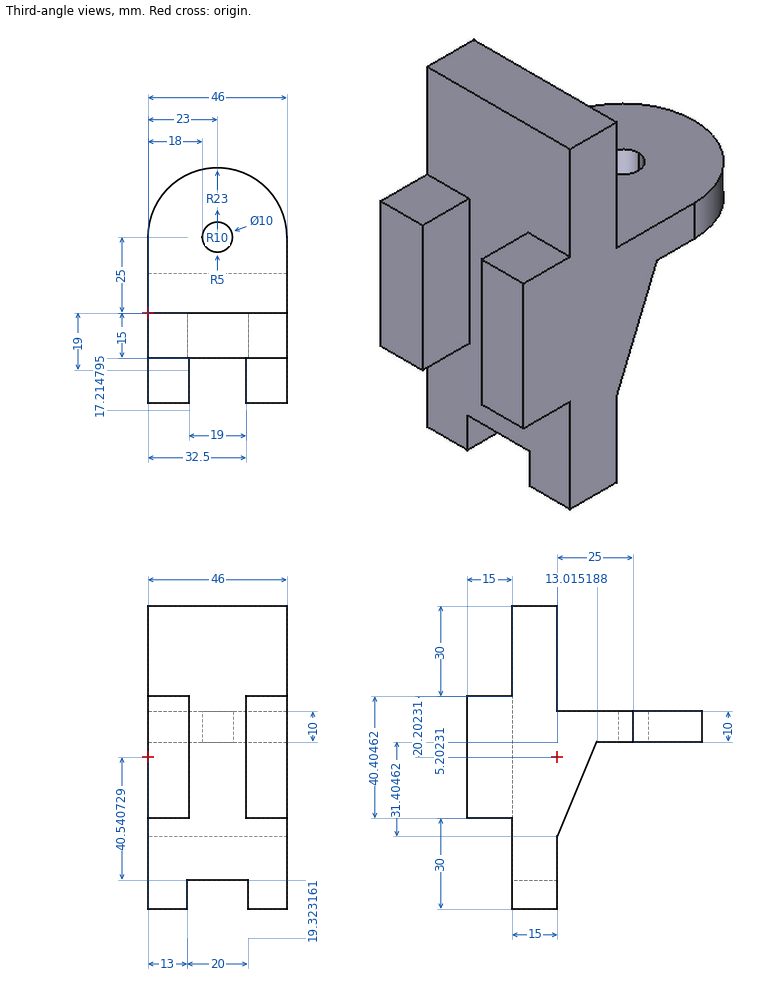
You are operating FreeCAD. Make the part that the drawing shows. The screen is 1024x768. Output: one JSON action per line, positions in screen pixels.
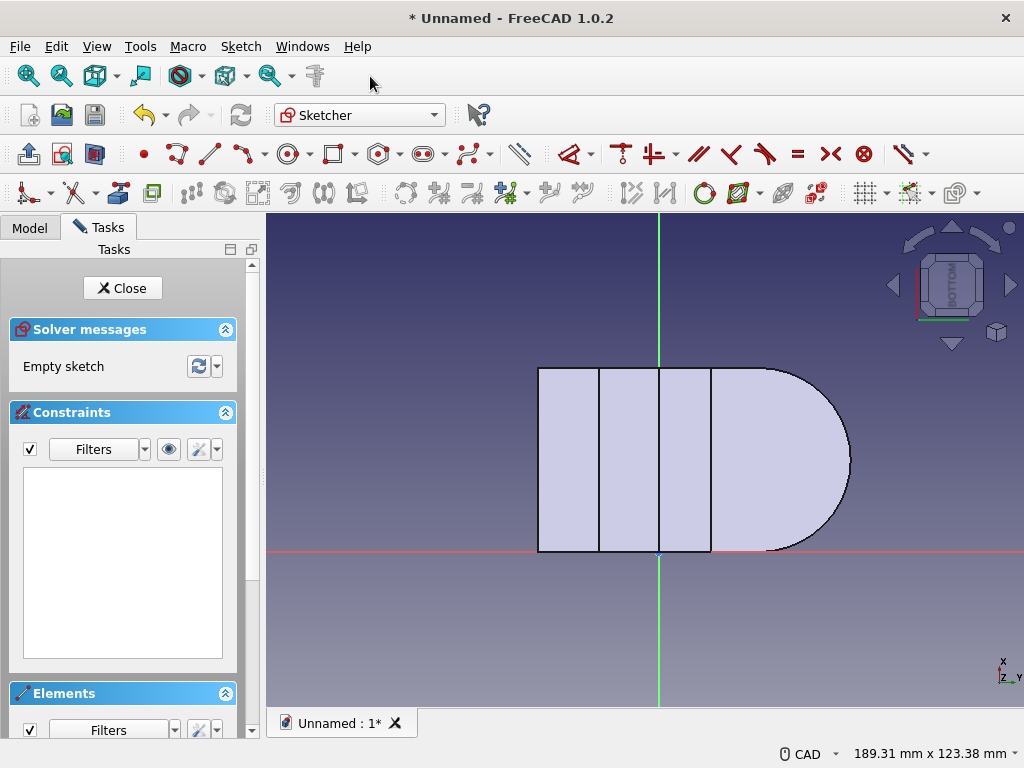
{"action": "key", "text": "q s"}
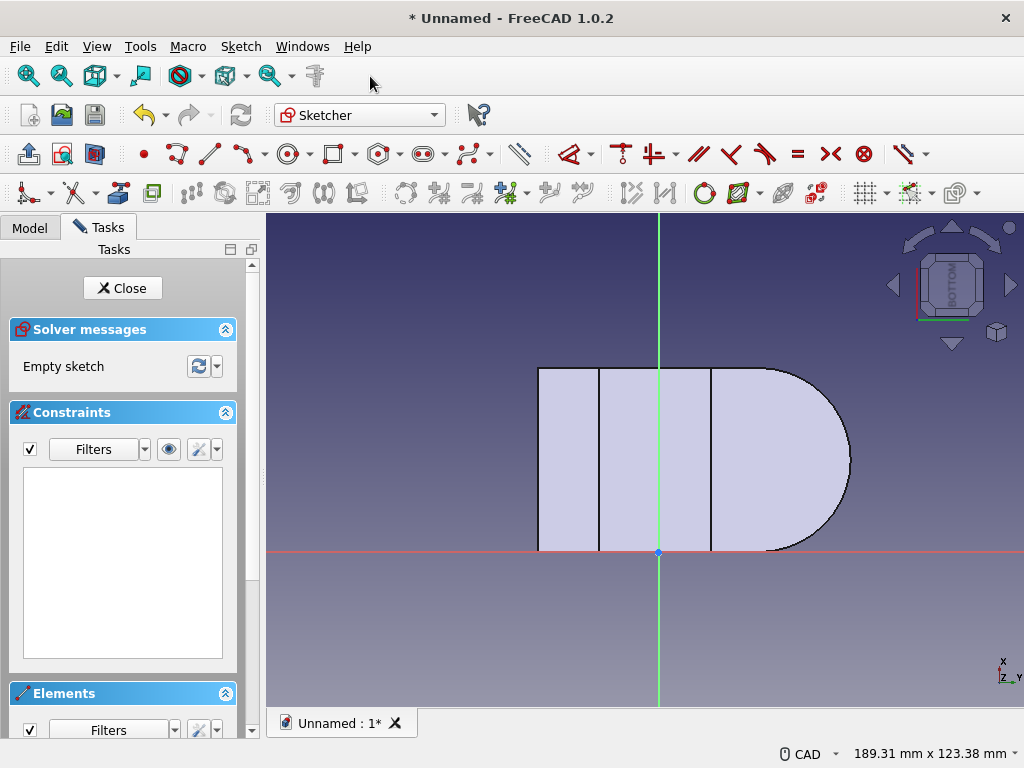
{"action": "scroll", "coordinate": [787, 460], "scroll_direction": "up", "scroll_amount": 10}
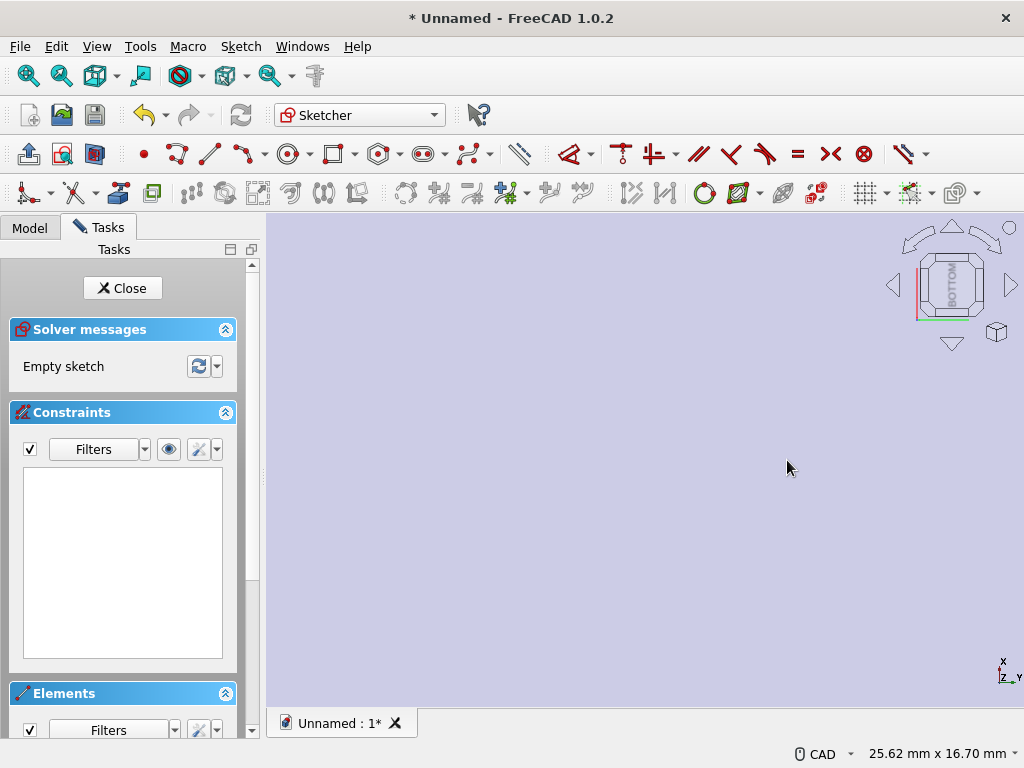
{"action": "key", "text": "g c"}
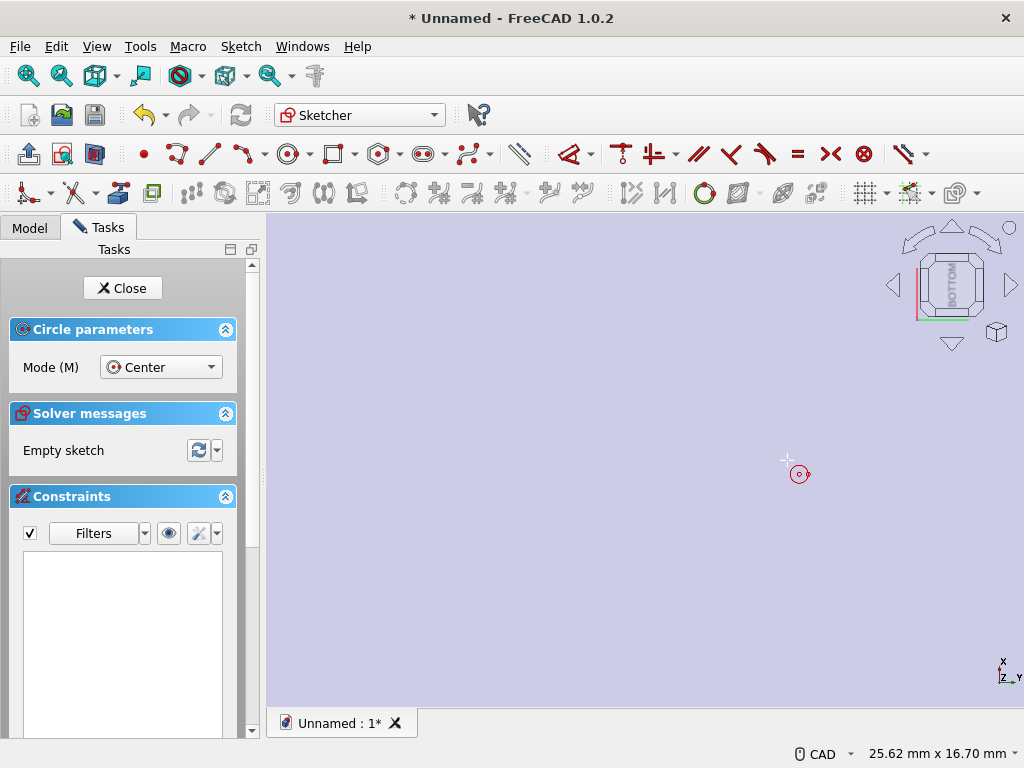
{"action": "left_click", "coordinate": [573, 457]}
{"action": "mouse_move", "coordinate": [678, 352]}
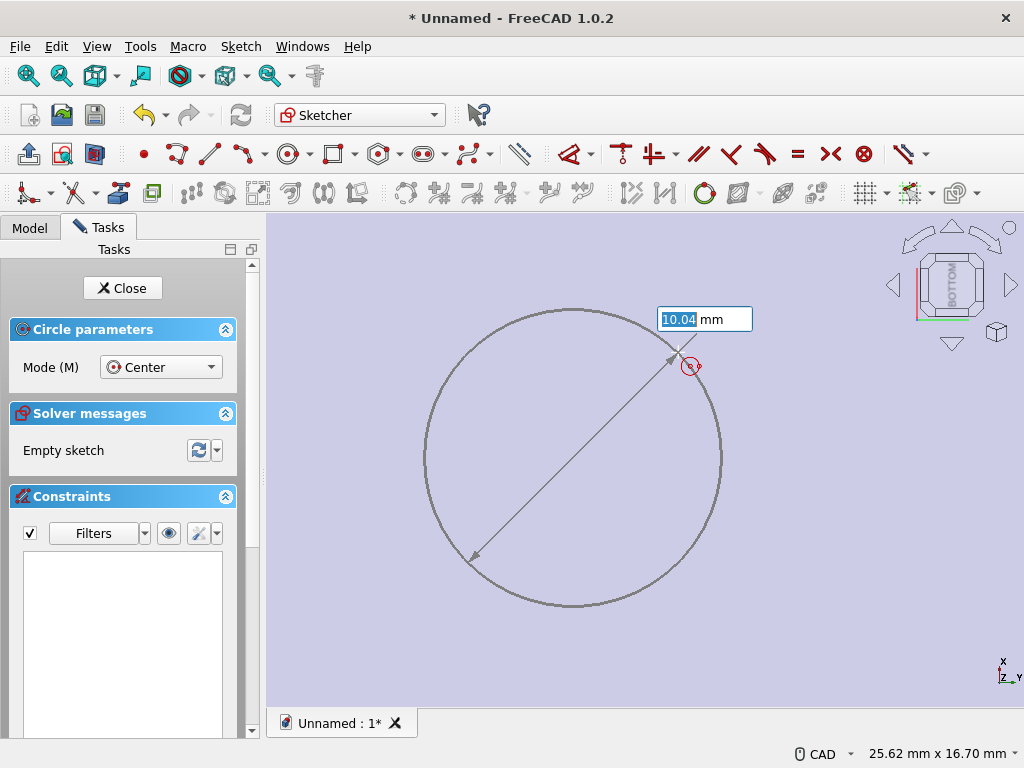
{"action": "type", "text": "10"}
{"action": "key", "text": "Return"}
{"action": "key", "text": "Escape"}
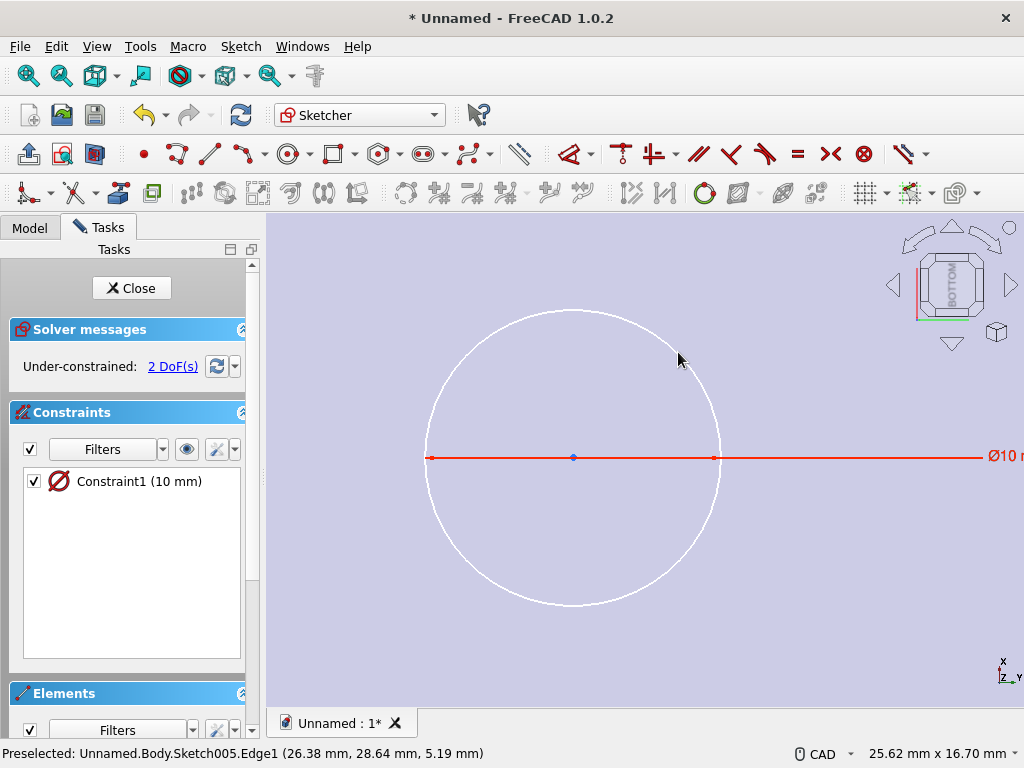
{"action": "left_click", "coordinate": [568, 154]}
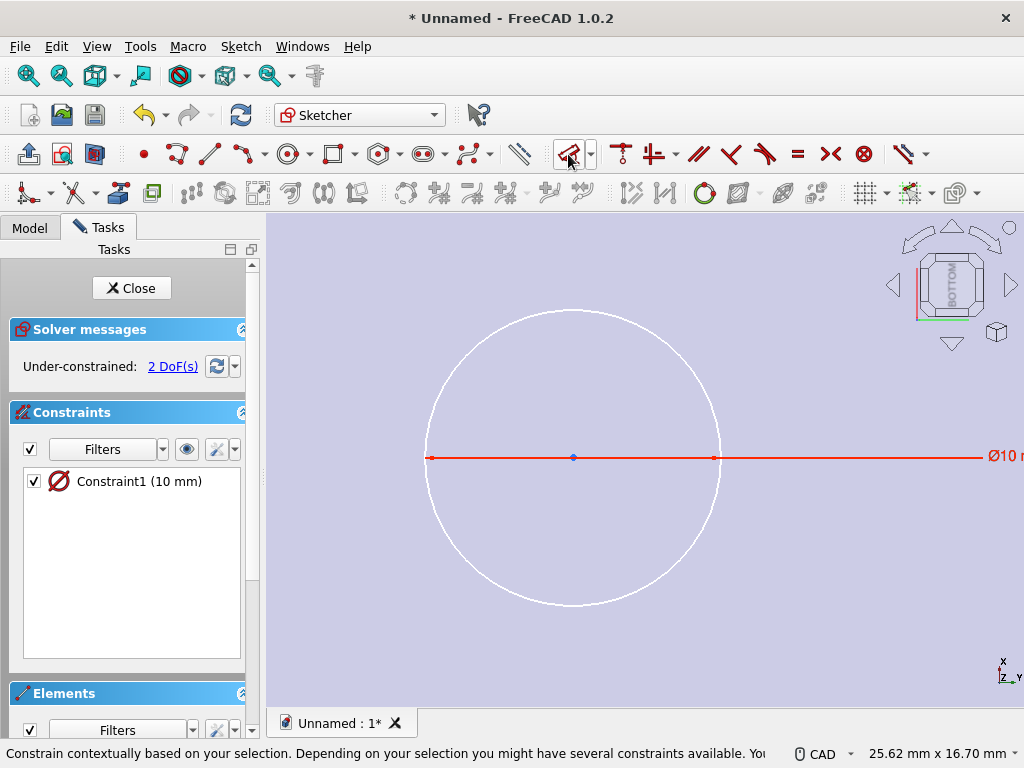
{"action": "left_click", "coordinate": [573, 458]}
{"action": "left_click", "coordinate": [369, 424]}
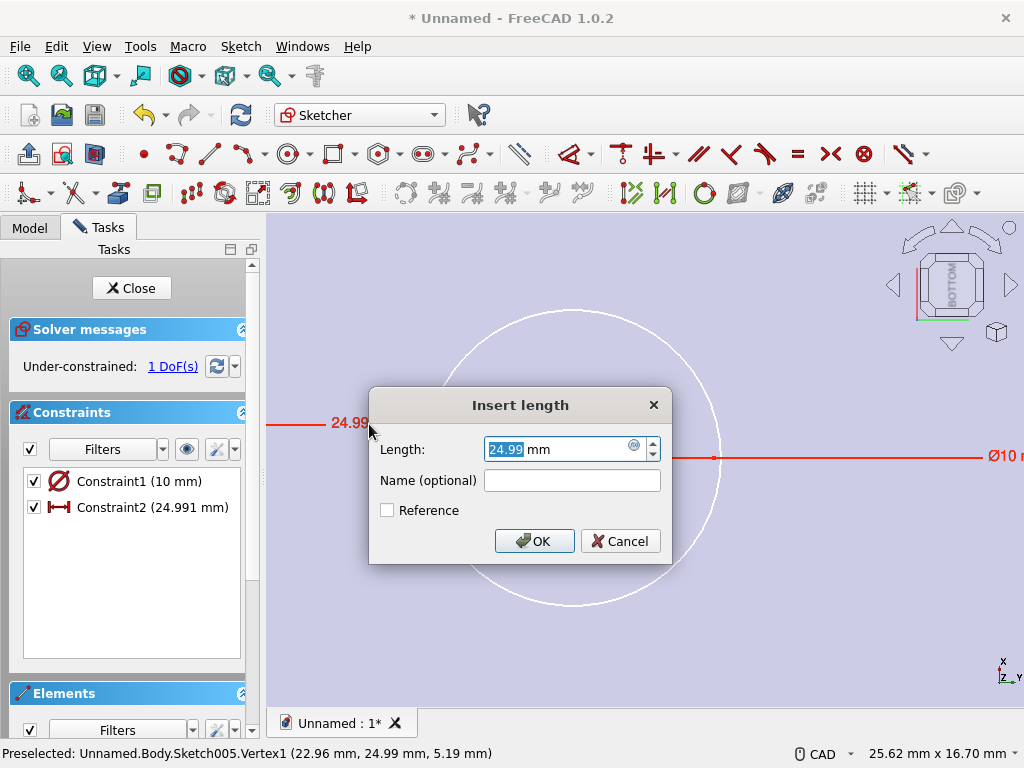
{"action": "type", "text": "25"}
{"action": "key", "text": "Return"}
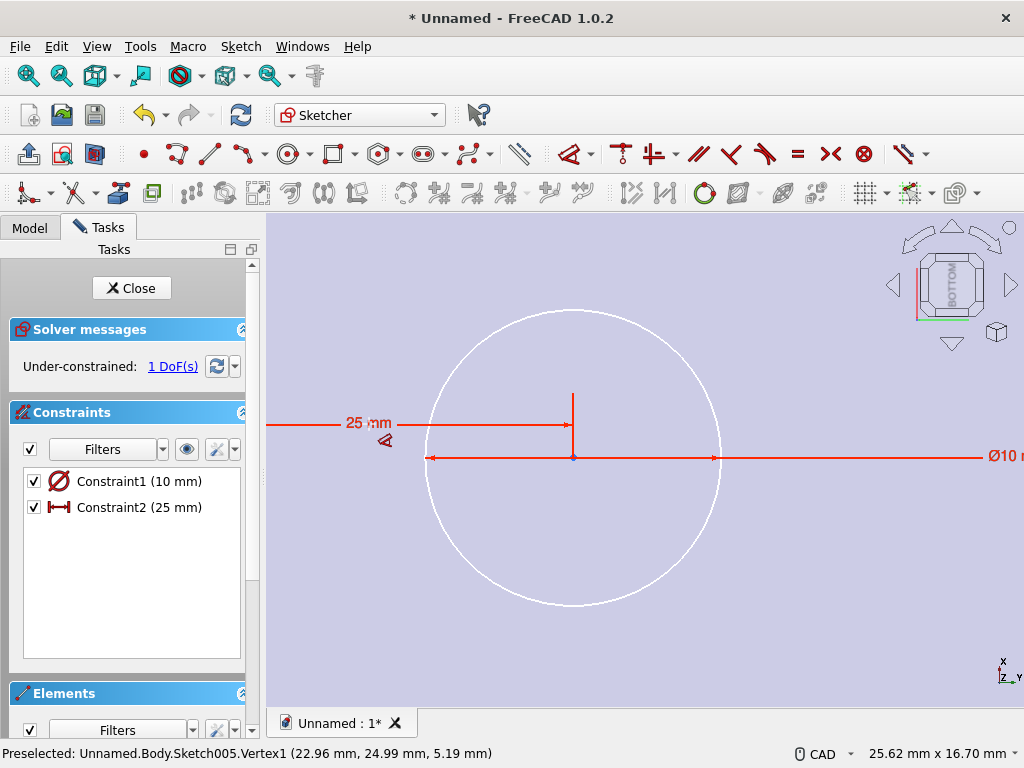
{"action": "left_click", "coordinate": [573, 458]}
{"action": "left_click", "coordinate": [607, 569]}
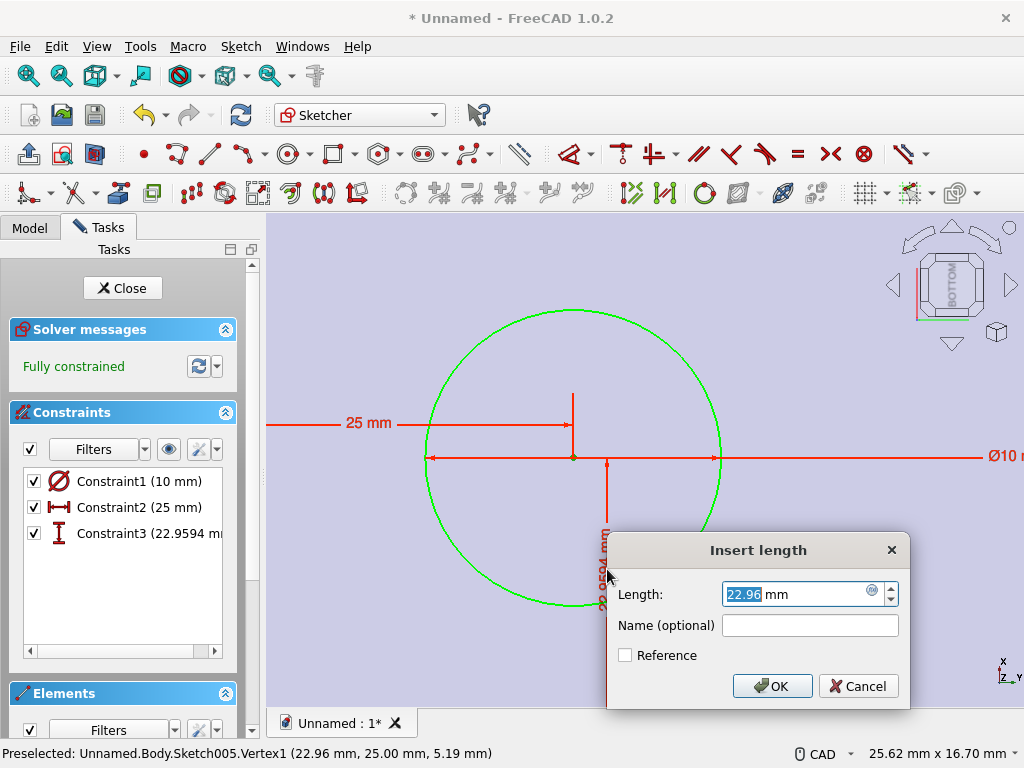
{"action": "type", "text": "23"}
{"action": "key", "text": "Return"}
{"action": "key", "text": "Escape"}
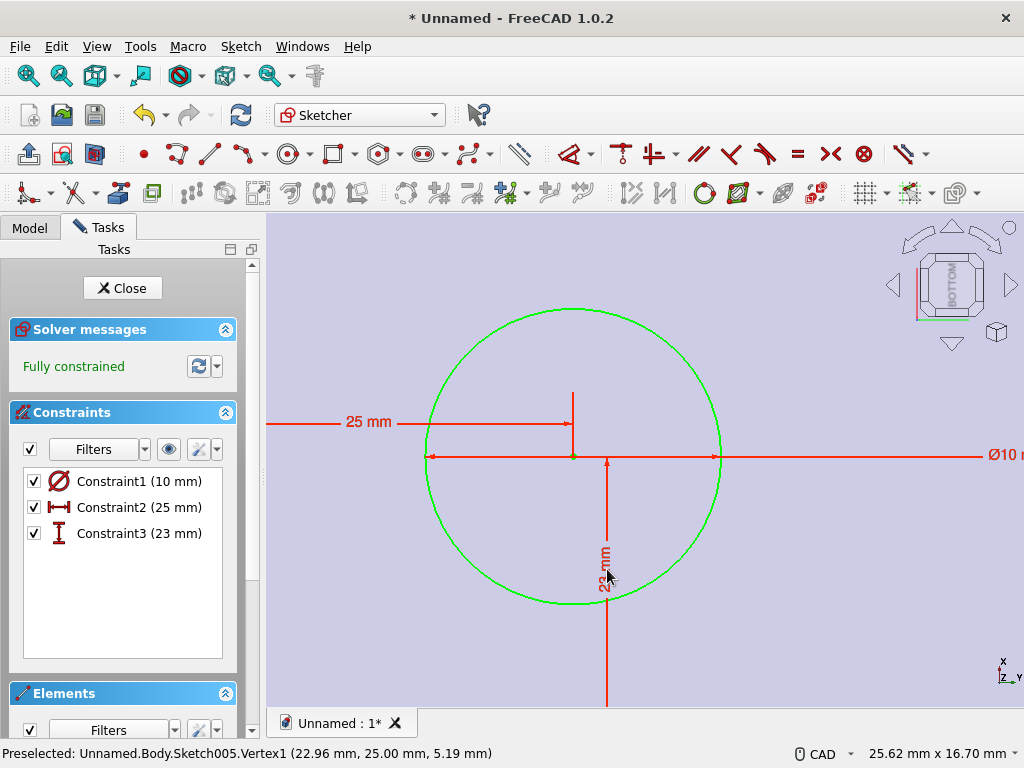
{"action": "left_click", "coordinate": [123, 288]}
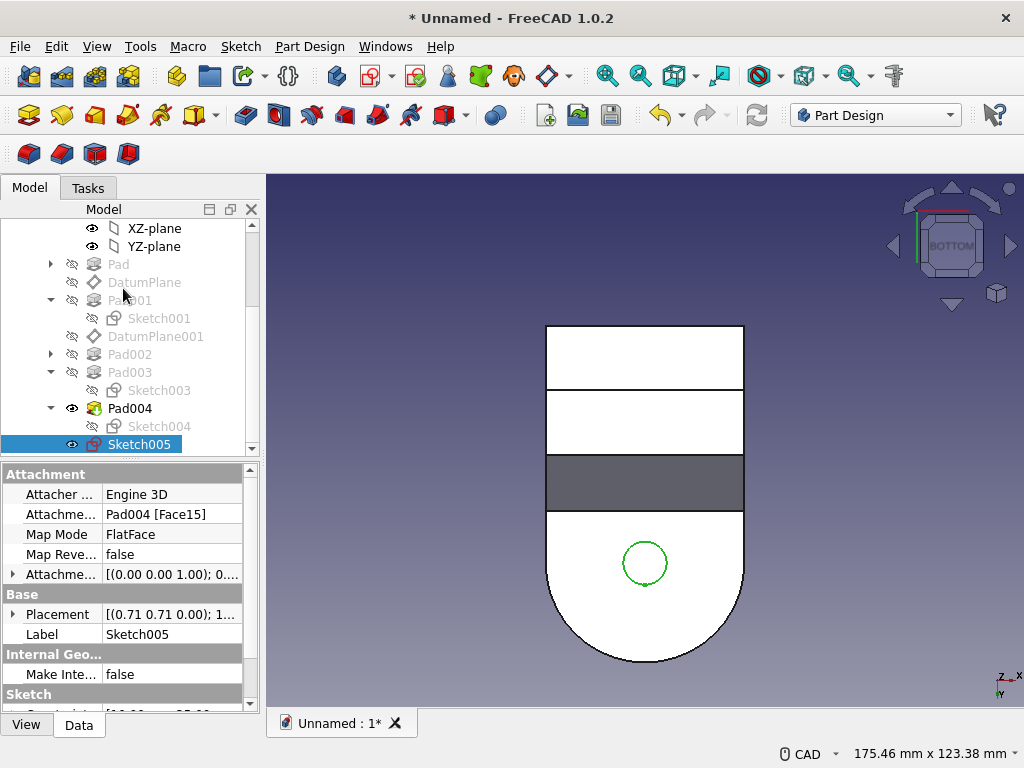
{"action": "left_click", "coordinate": [246, 116]}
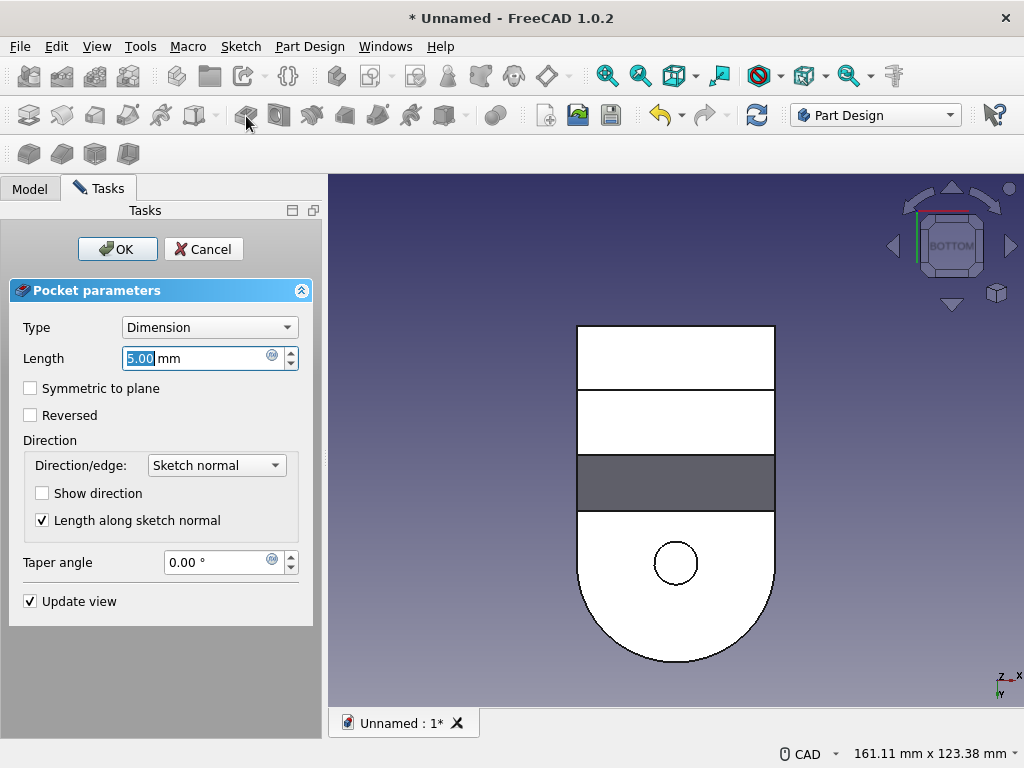
{"action": "type", "text": "10"}
{"action": "key", "text": "Tab"}